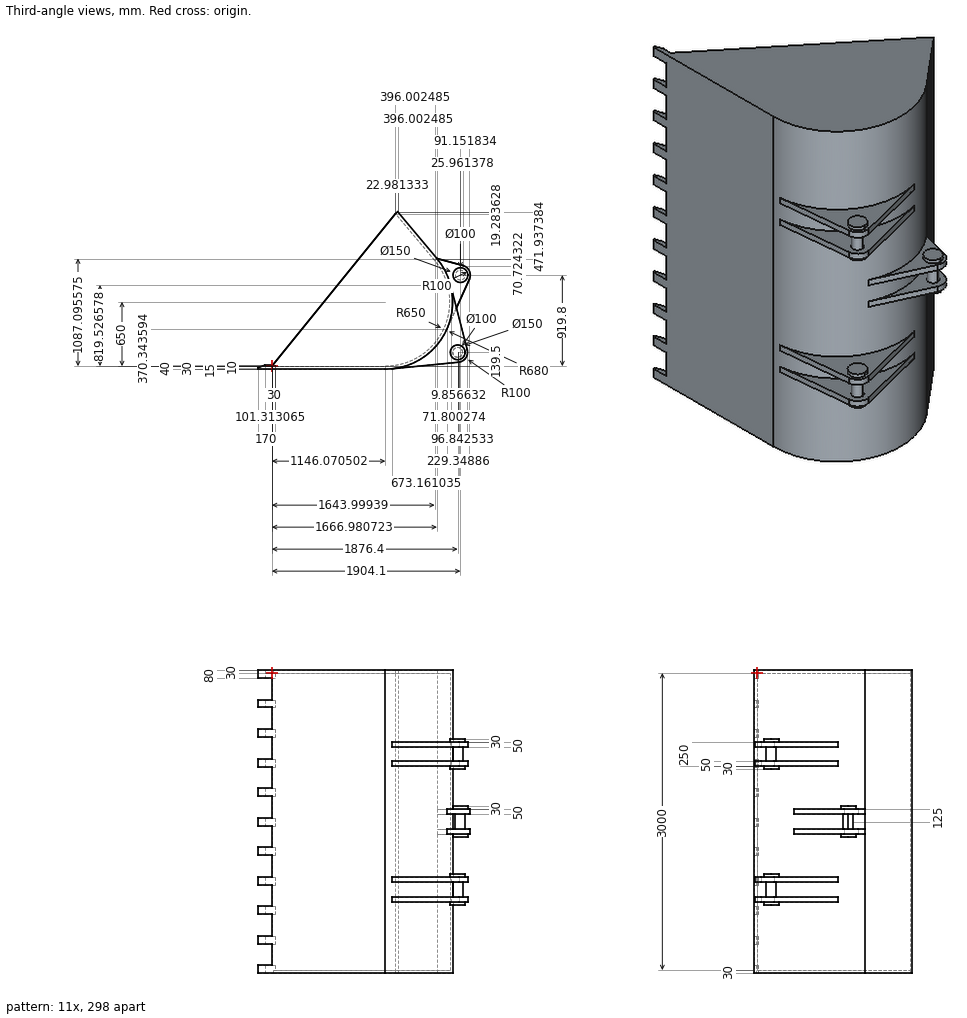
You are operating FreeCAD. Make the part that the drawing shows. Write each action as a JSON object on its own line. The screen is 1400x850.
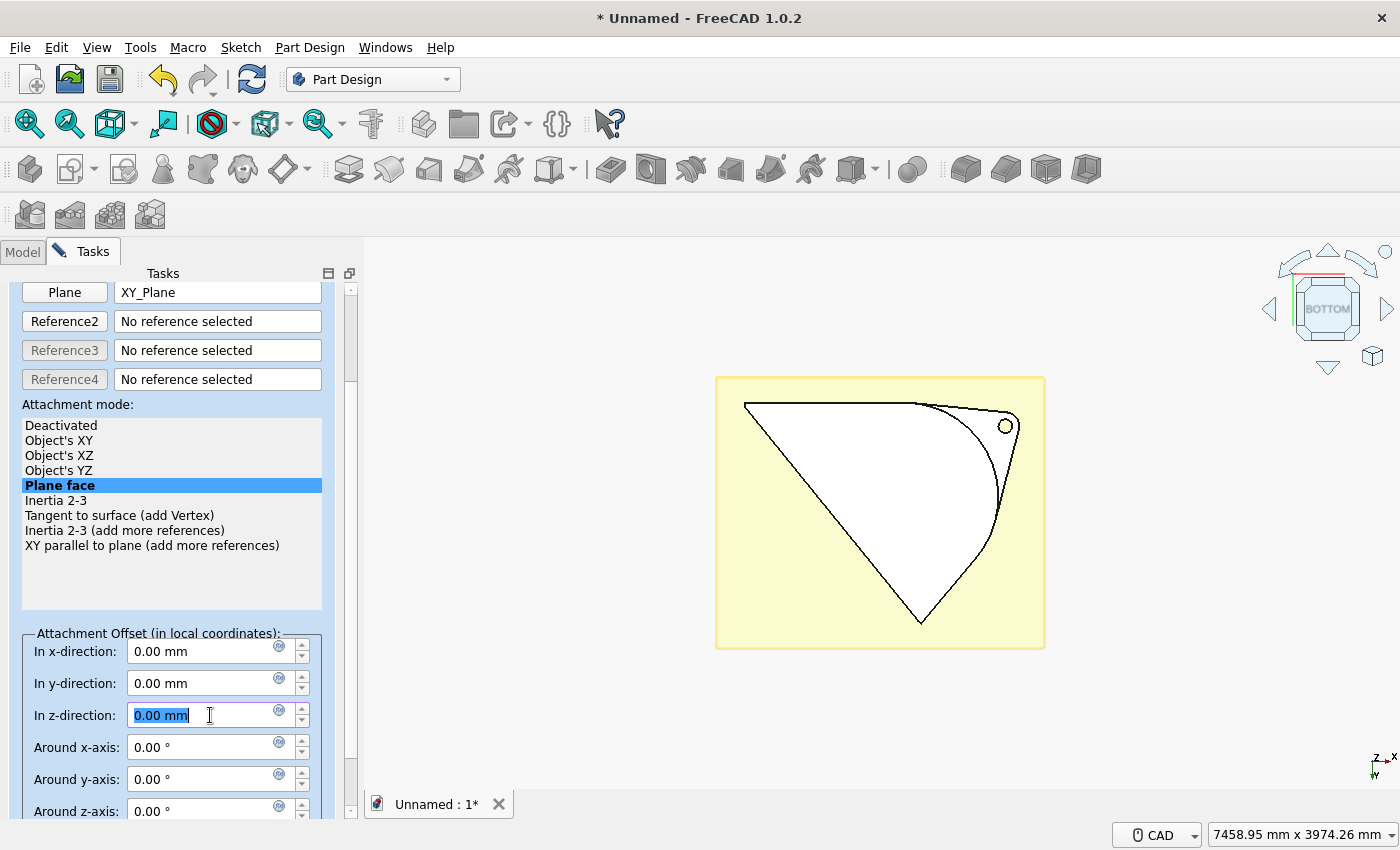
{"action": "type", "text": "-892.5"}
{"action": "key", "text": "Tab"}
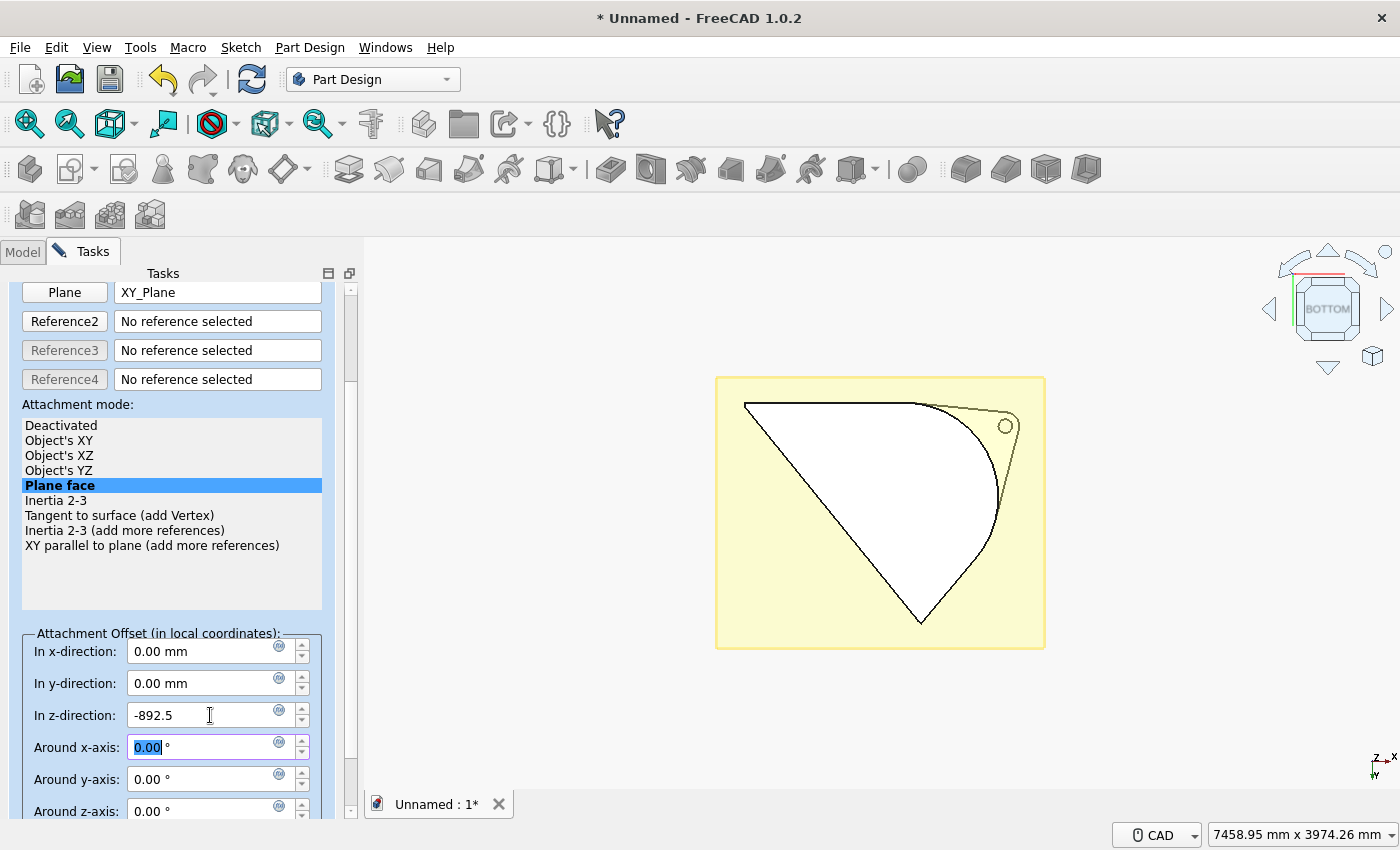
{"action": "scroll", "coordinate": [351, 550], "scroll_direction": "up", "scroll_amount": 3}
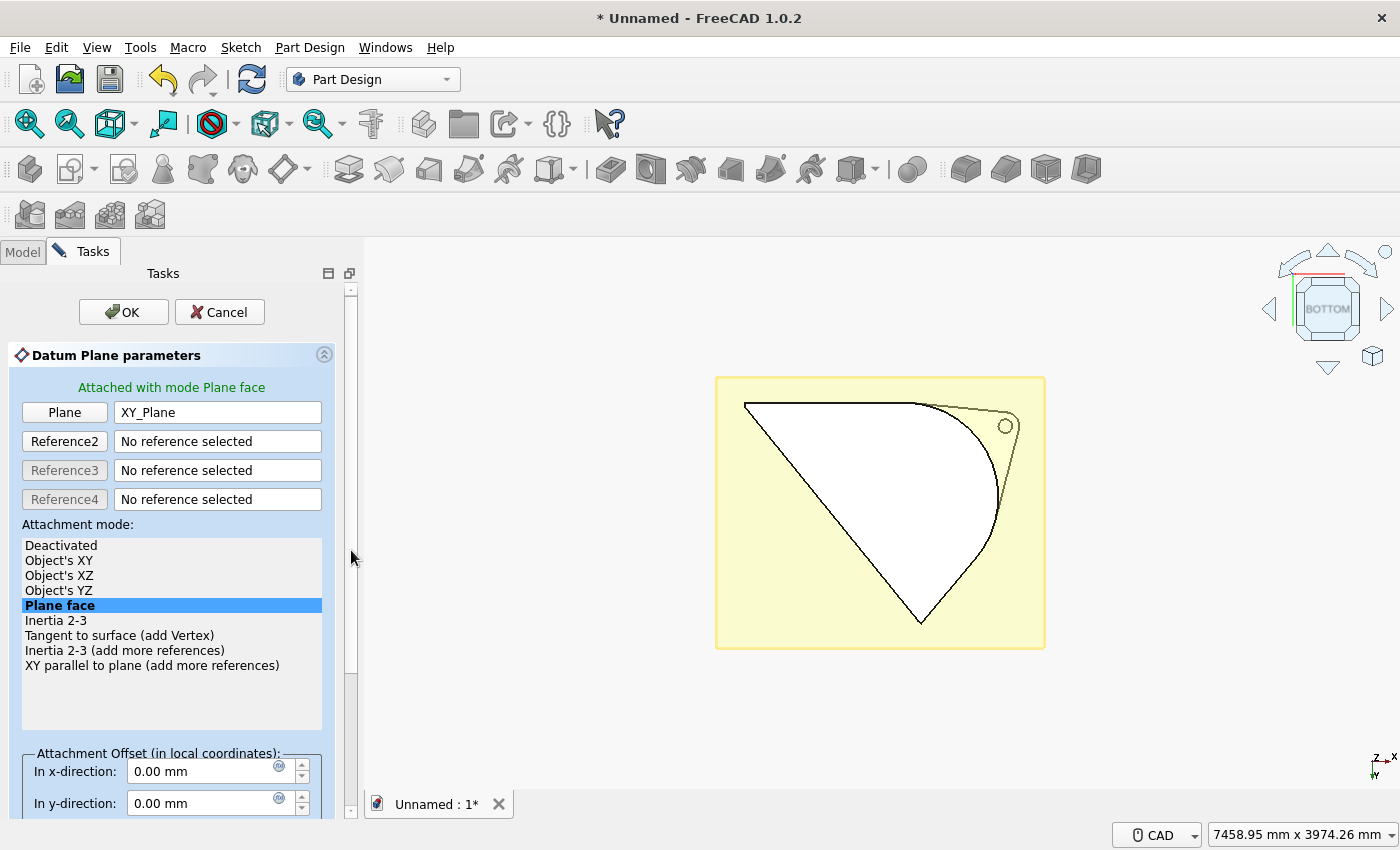
{"action": "left_click", "coordinate": [124, 312]}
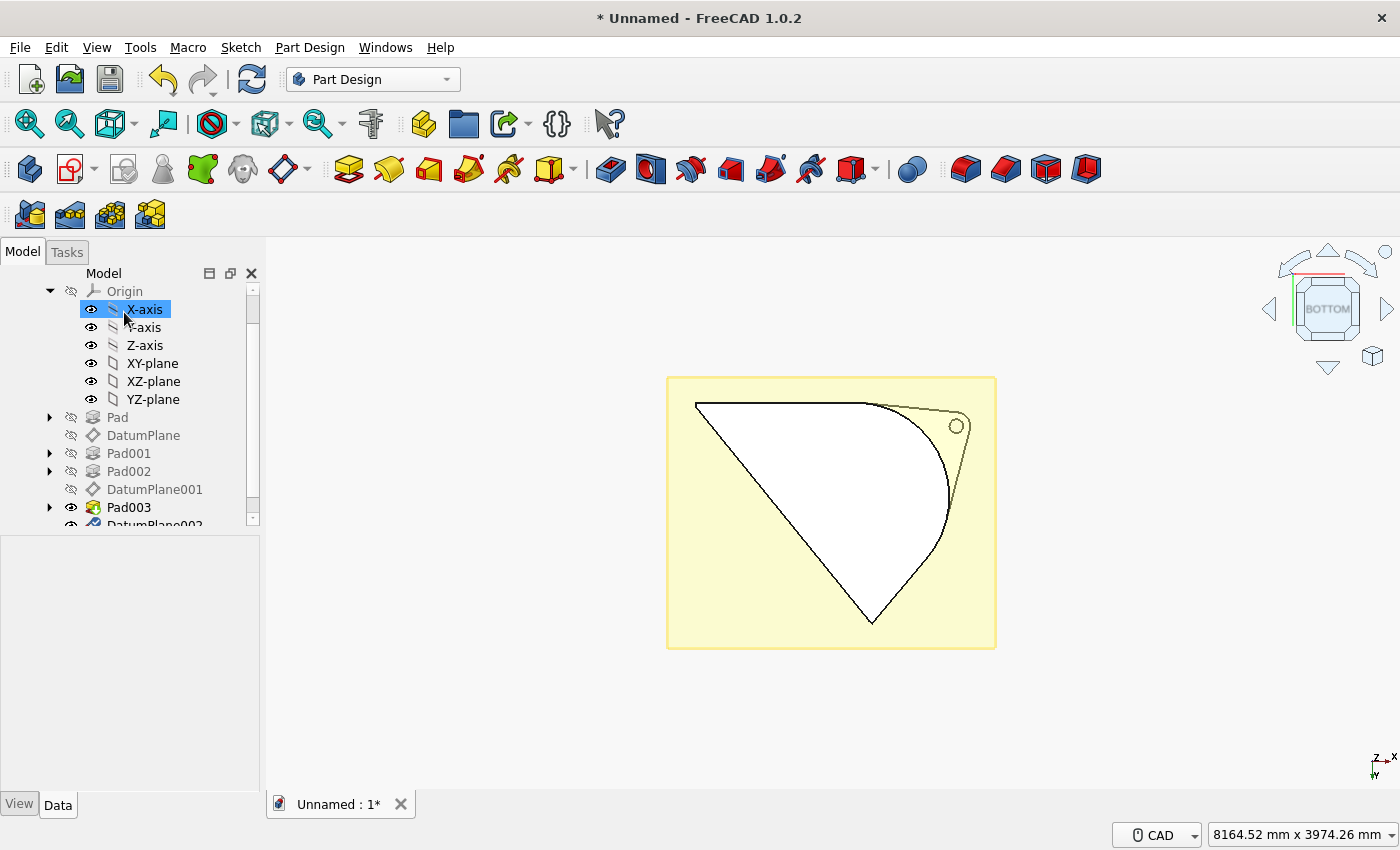
{"action": "left_click", "coordinate": [116, 525]}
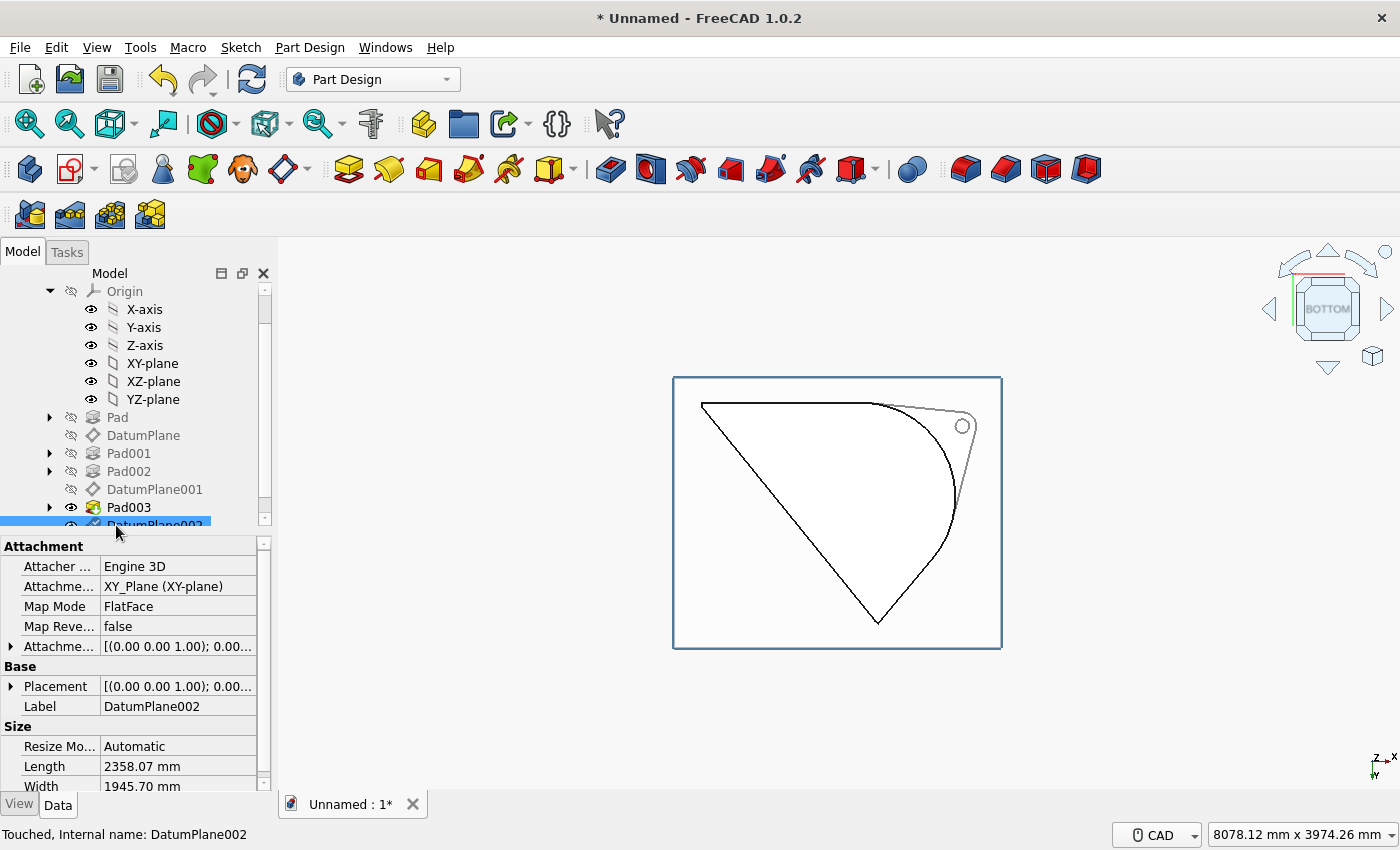
{"action": "left_click", "coordinate": [70, 170]}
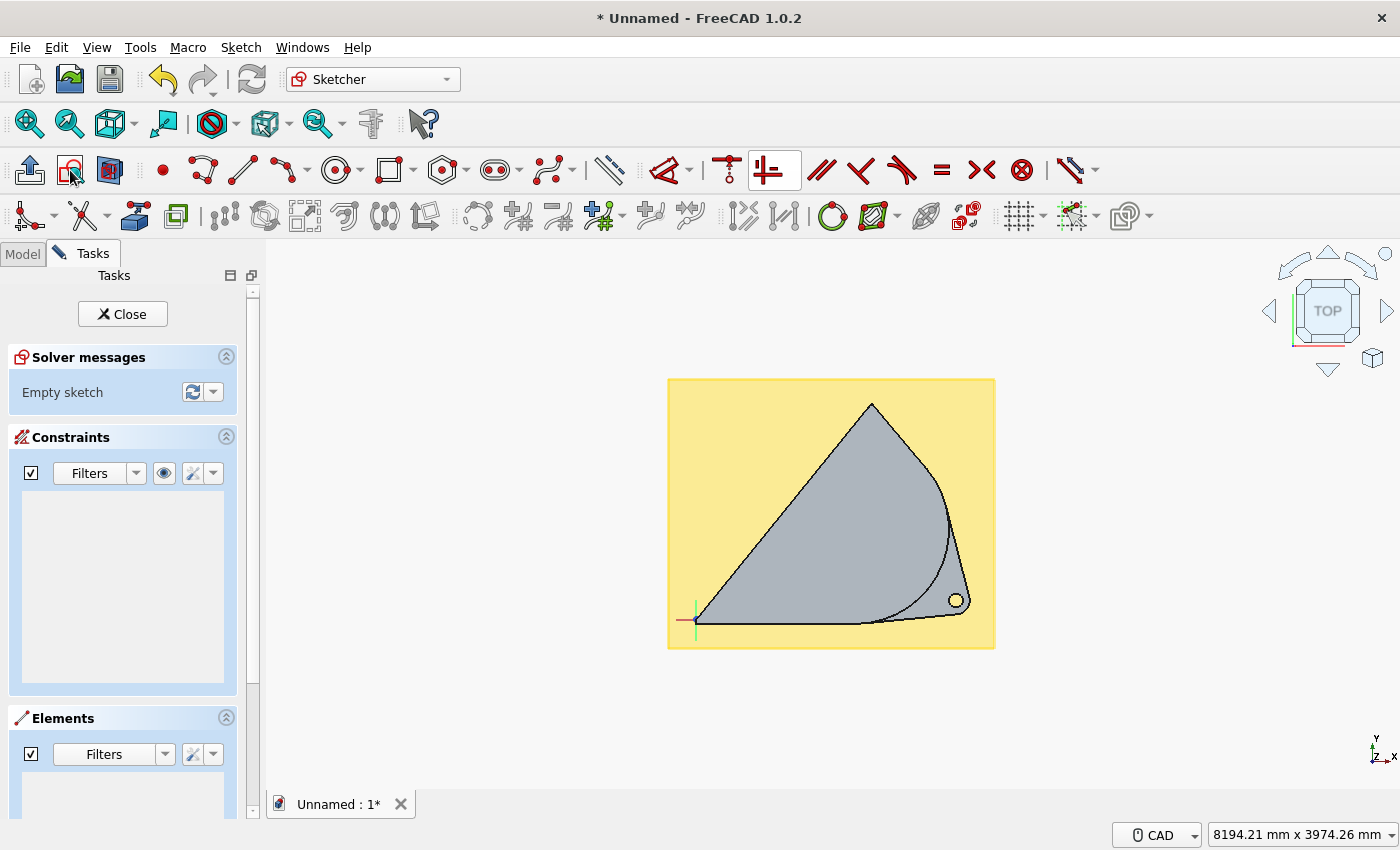
{"action": "left_click", "coordinate": [110, 170]}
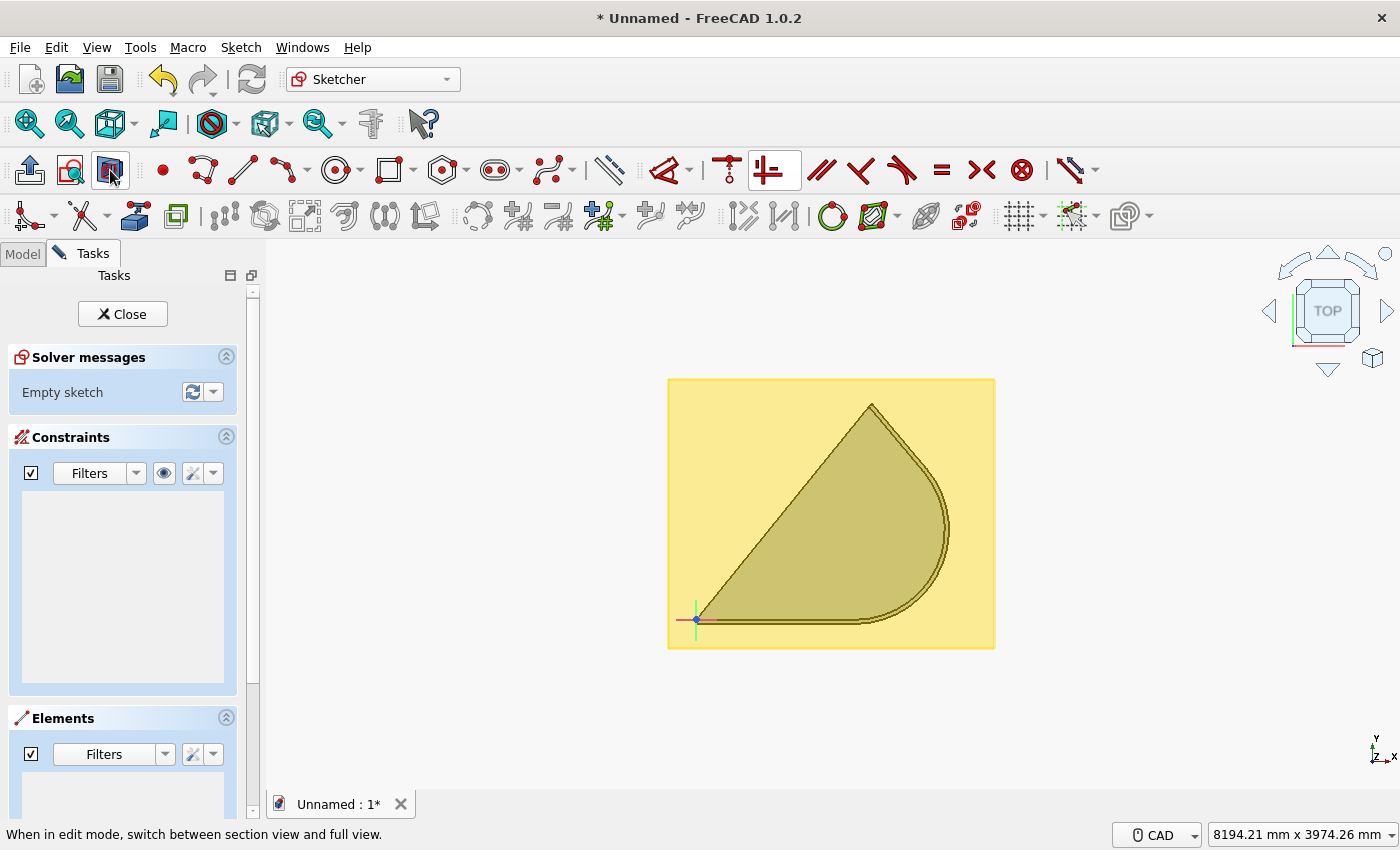
{"action": "scroll", "coordinate": [888, 607], "scroll_direction": "up", "scroll_amount": 4}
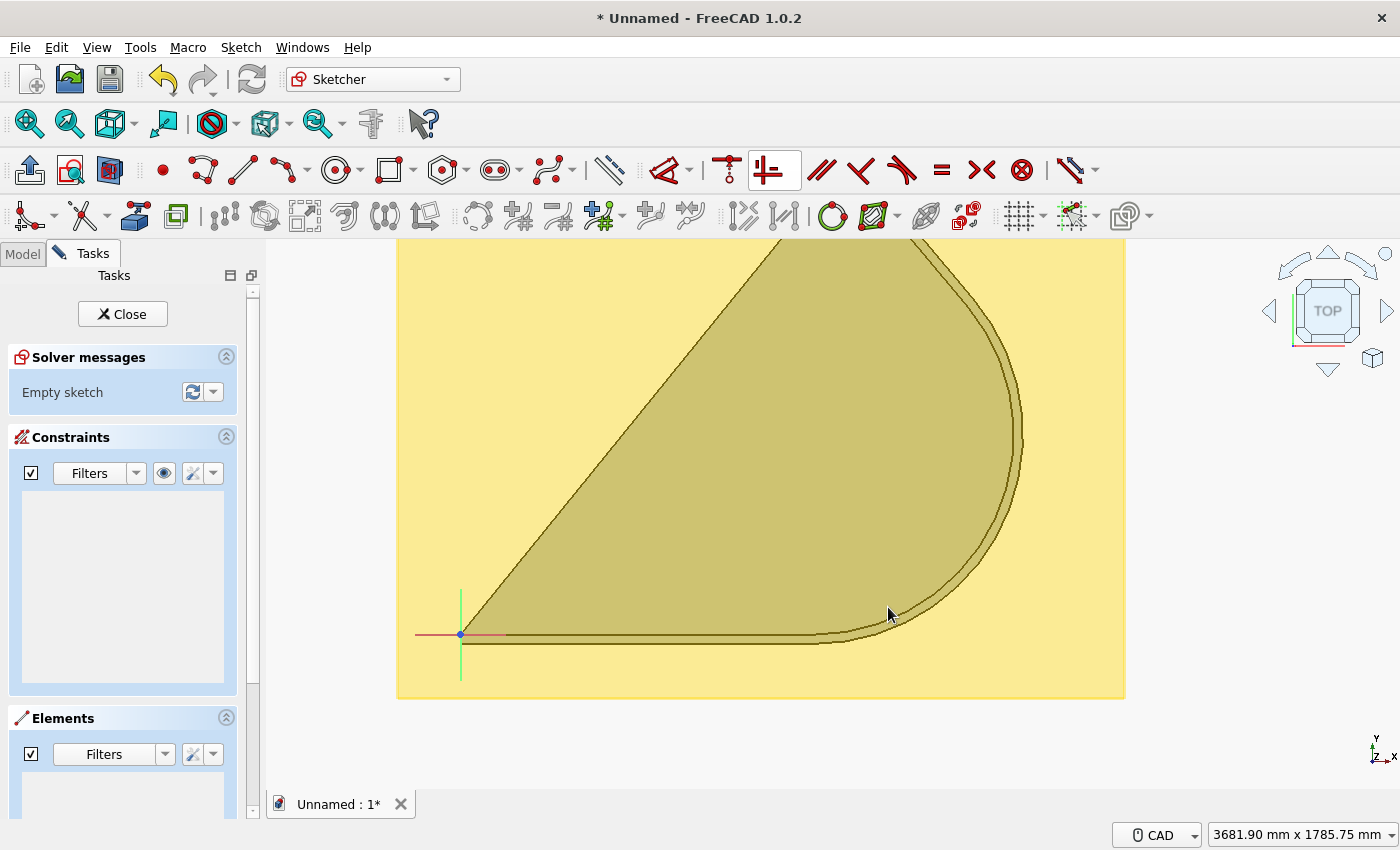
{"action": "left_click", "coordinate": [244, 170]}